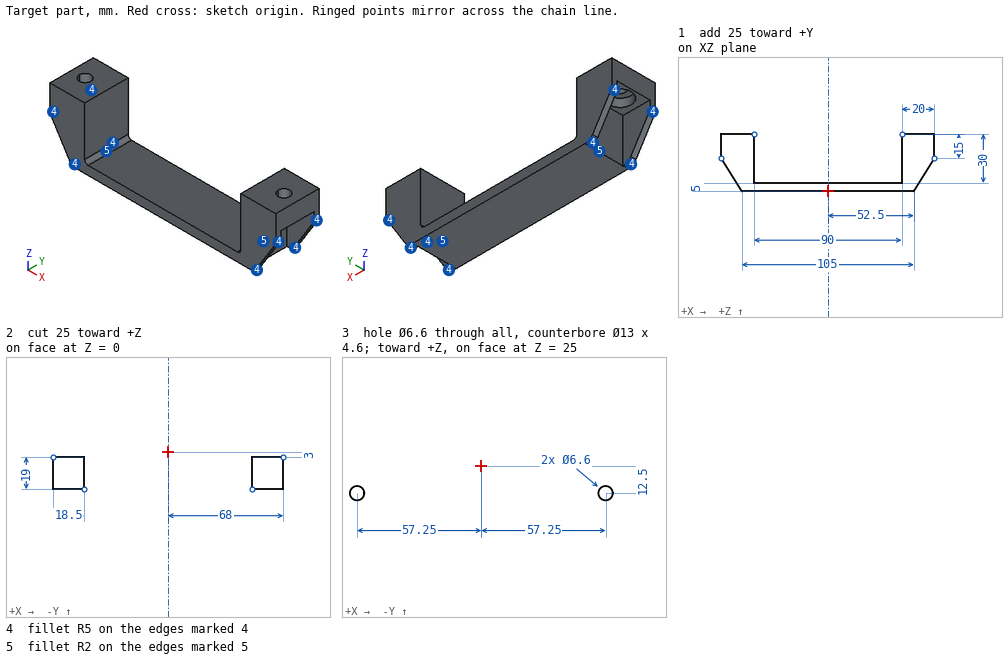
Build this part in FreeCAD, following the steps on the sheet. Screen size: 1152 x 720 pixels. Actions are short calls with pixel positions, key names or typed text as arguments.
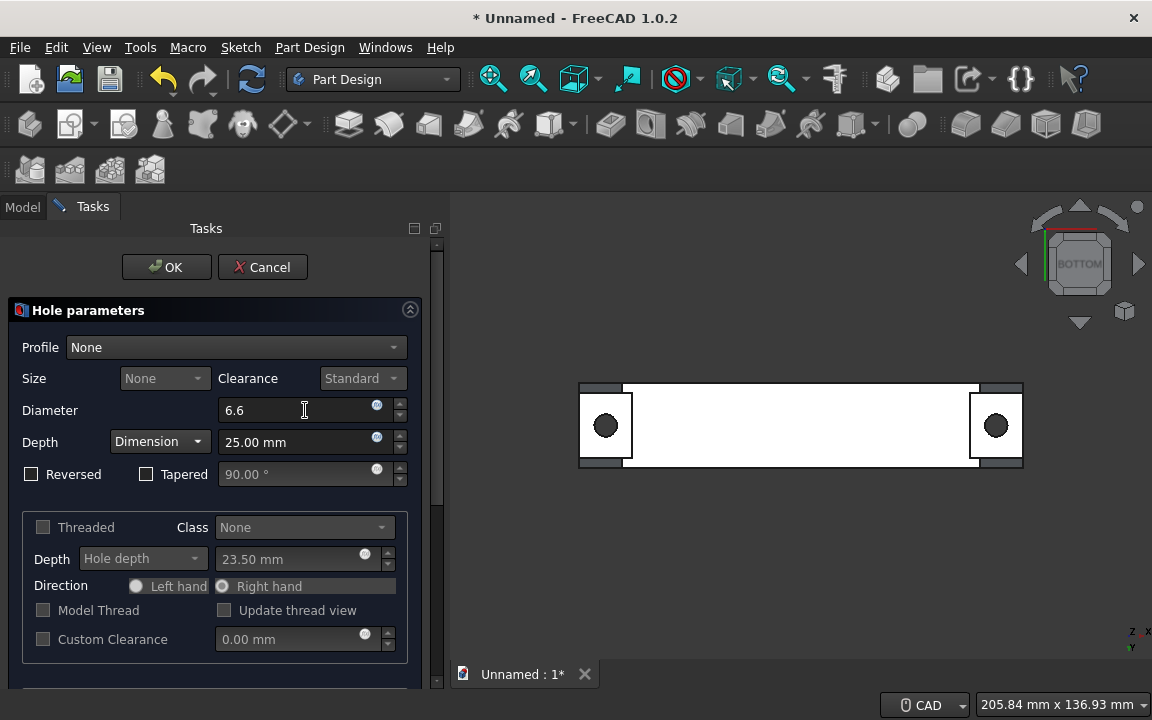
click(161, 442)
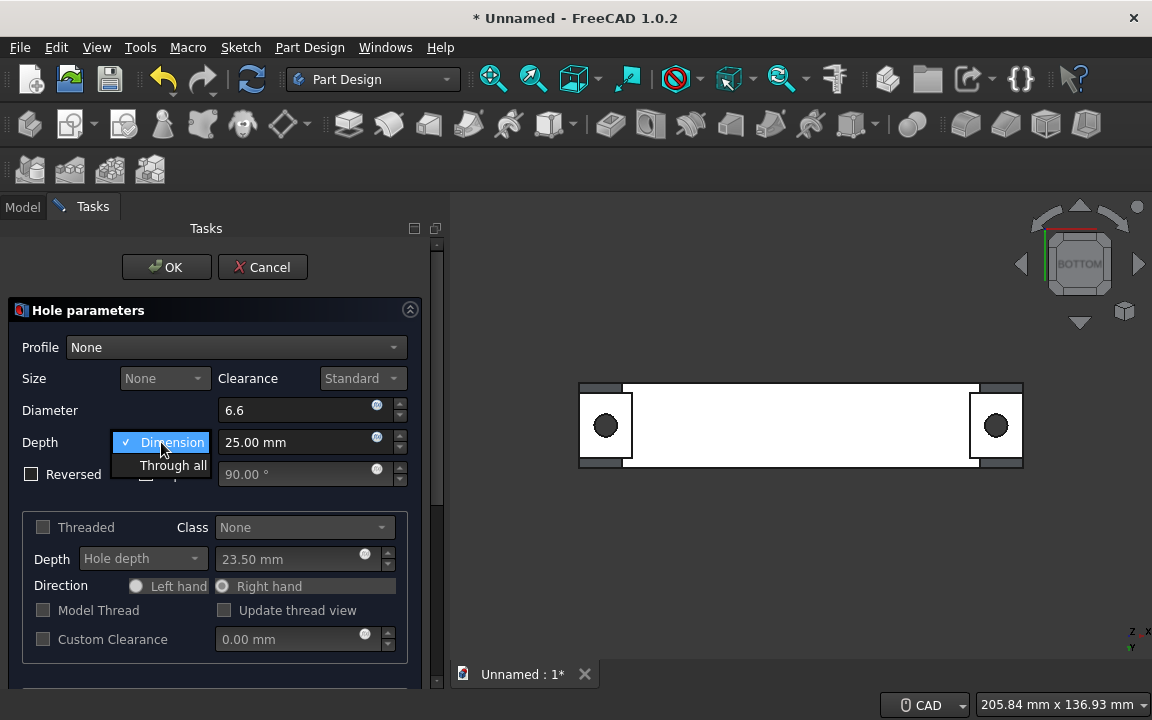
click(160, 466)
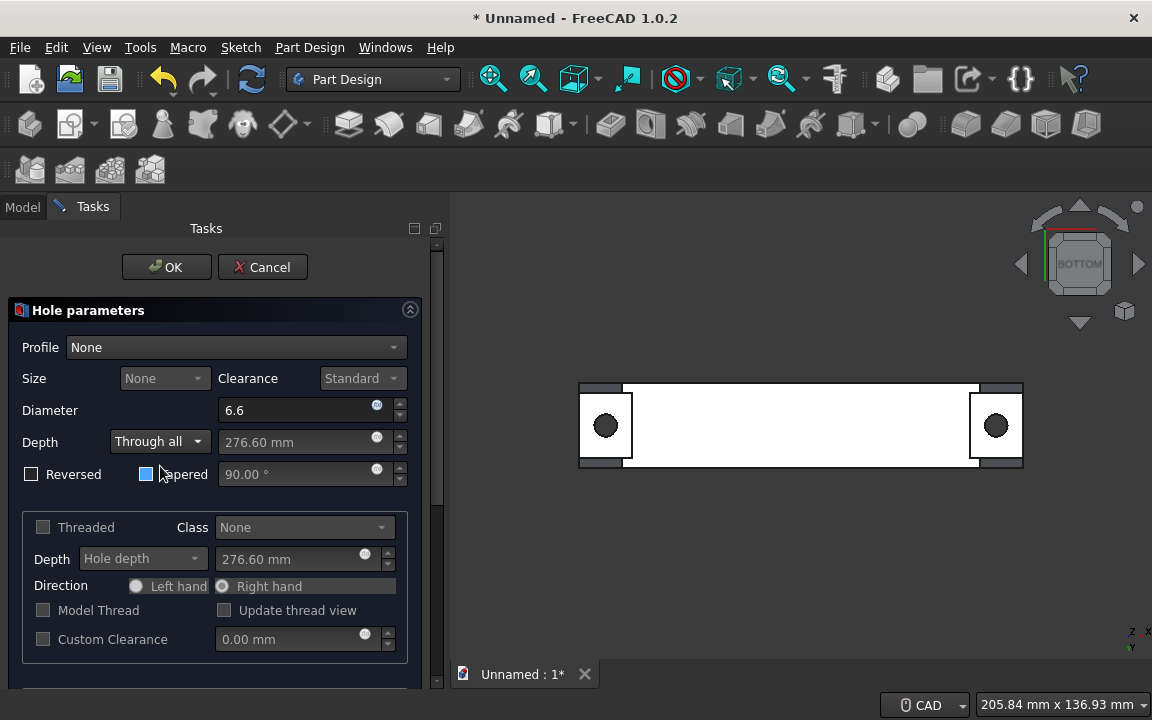
scroll(437, 463, down, 2)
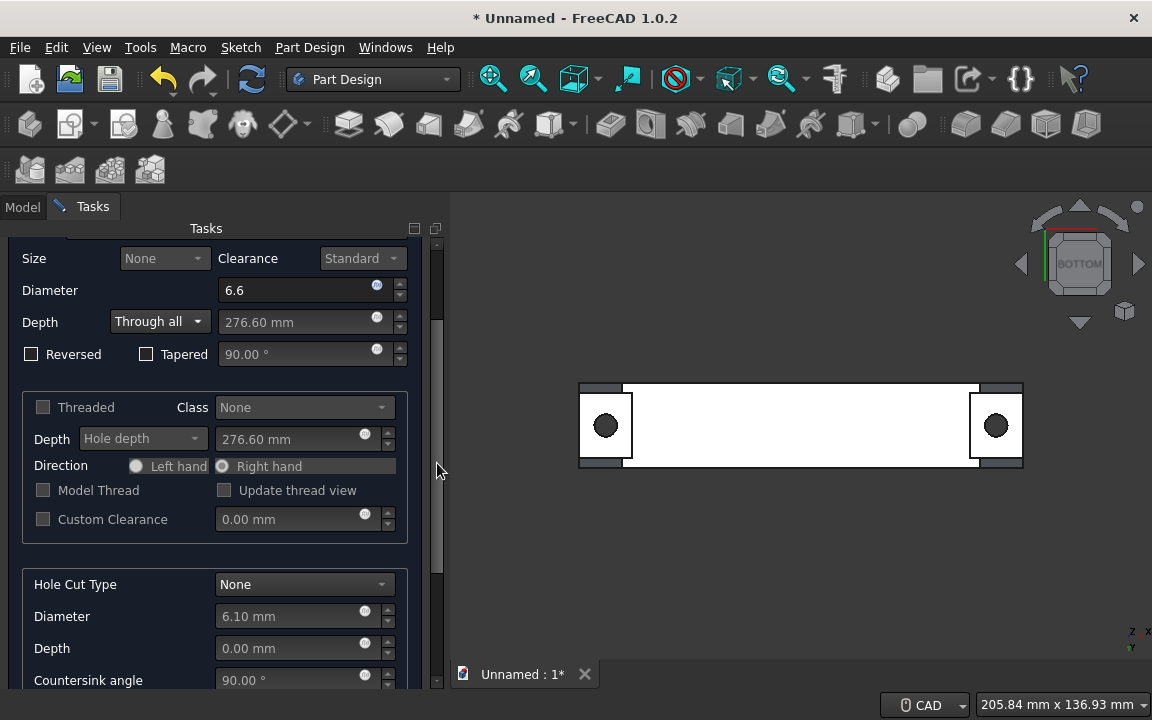
click(306, 584)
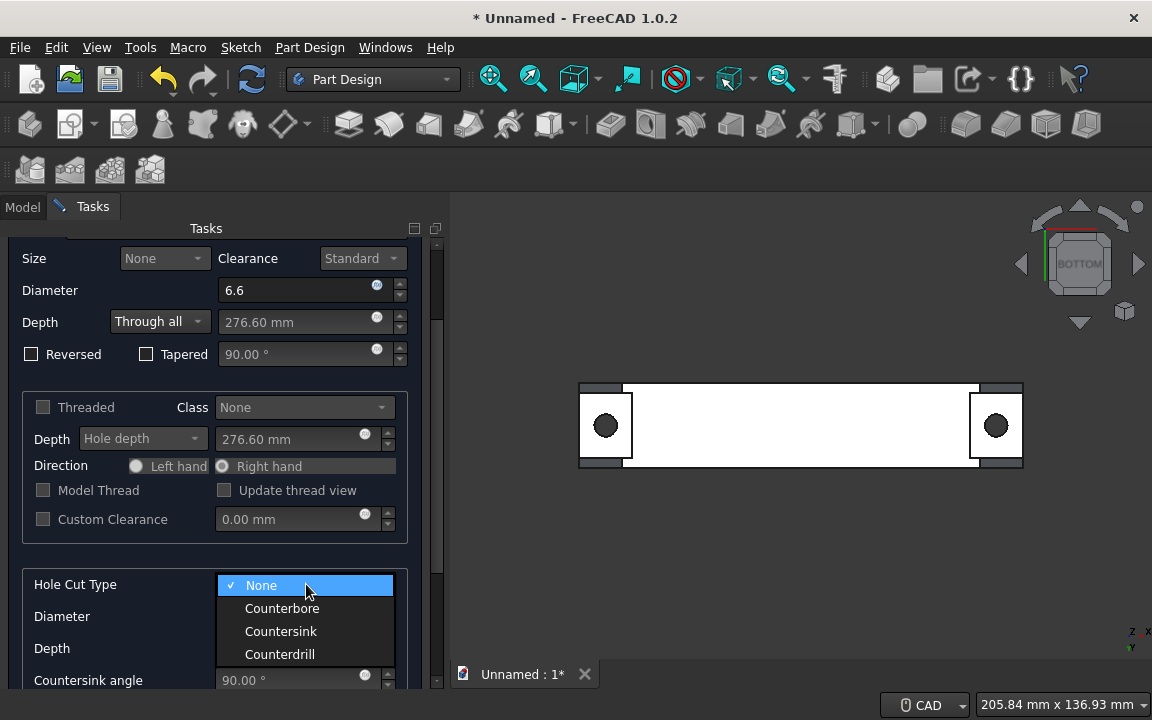
click(304, 608)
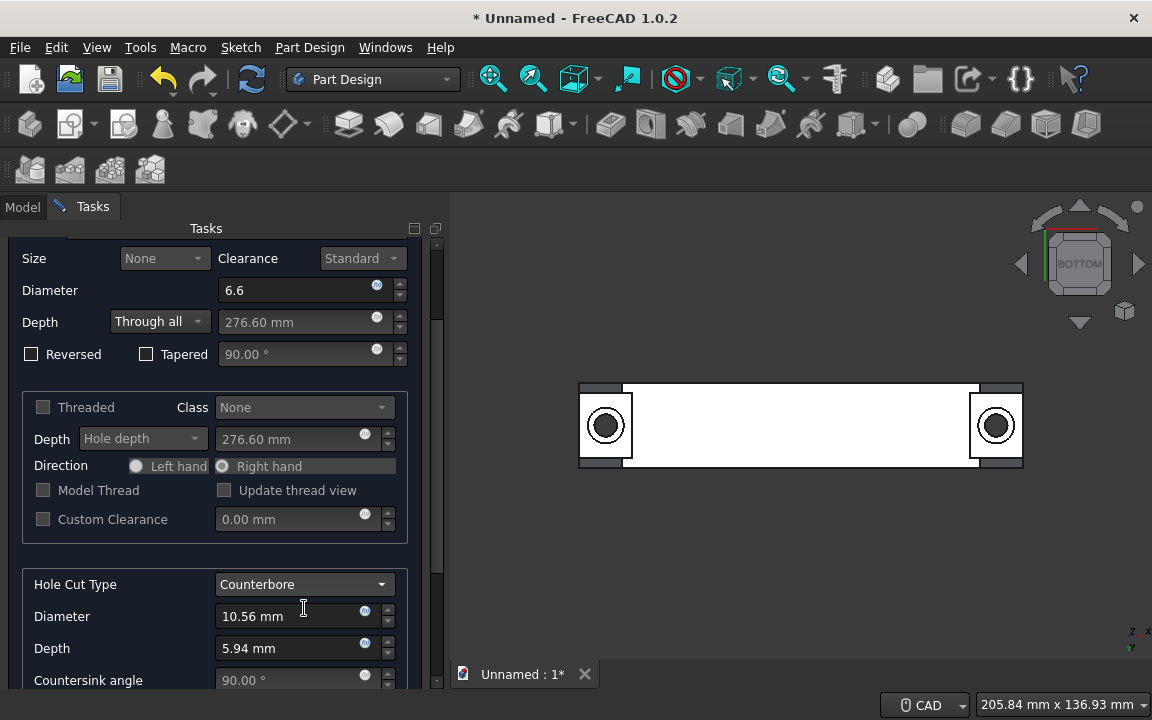
triple_click(298, 616)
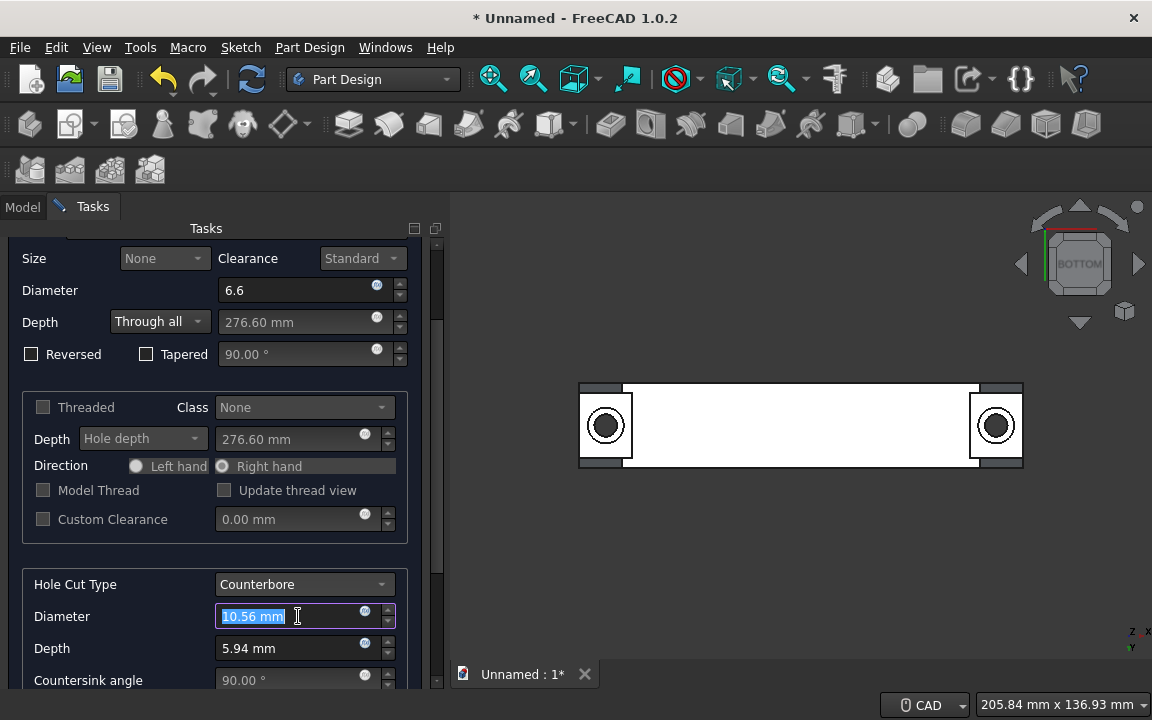
text(13)
key(Tab)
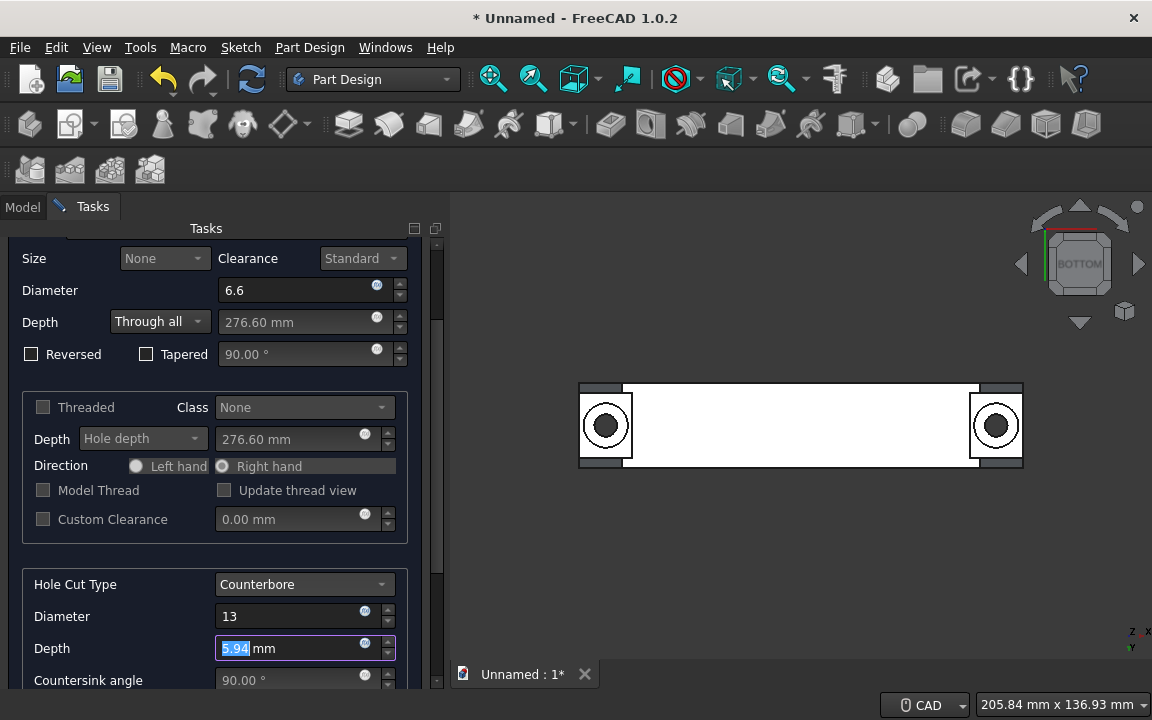
text(4.6)
key(Tab)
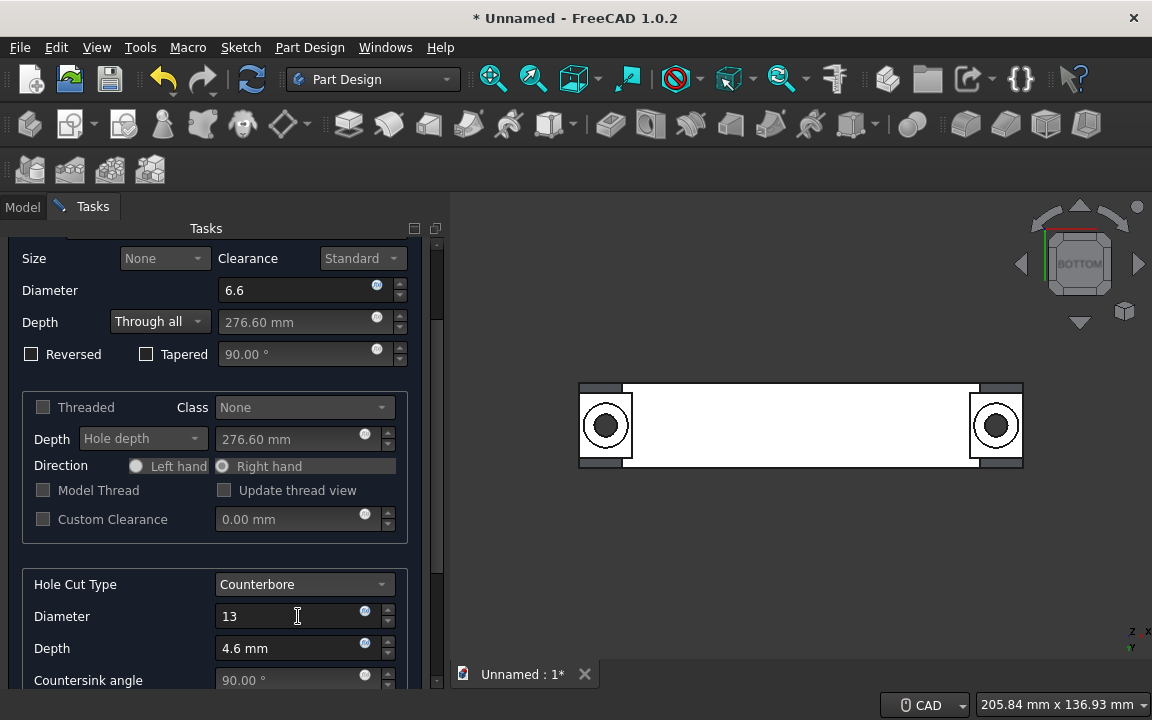
scroll(437, 463, up, 3)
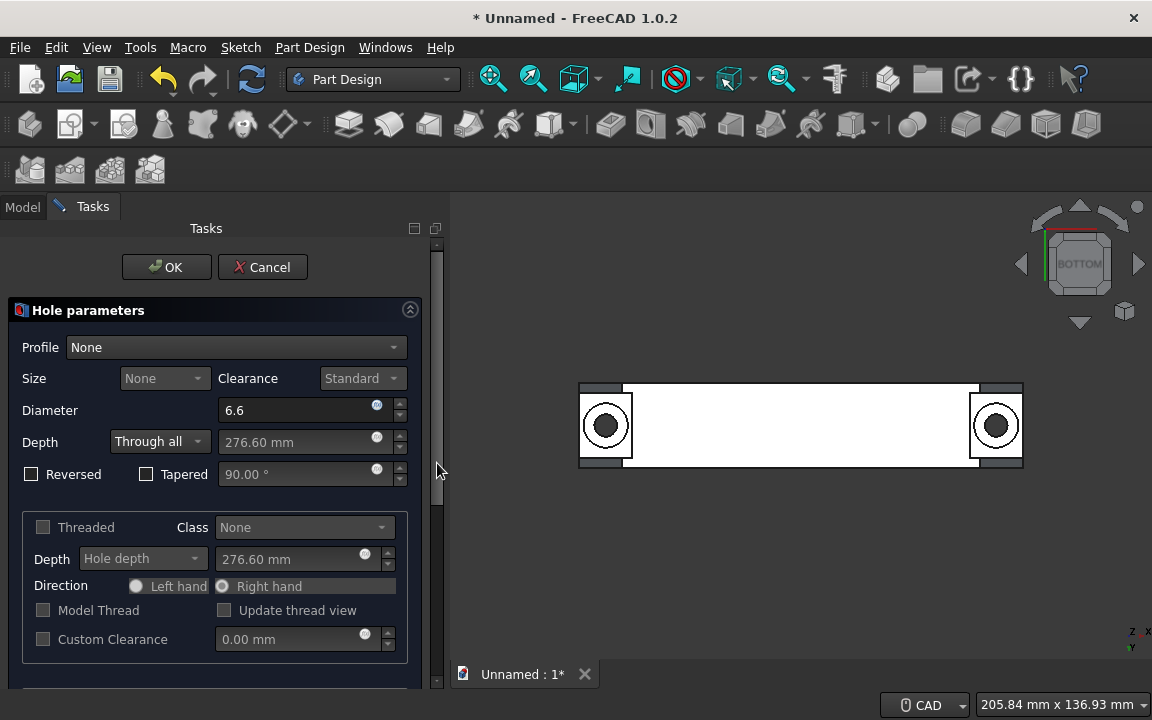
click(167, 267)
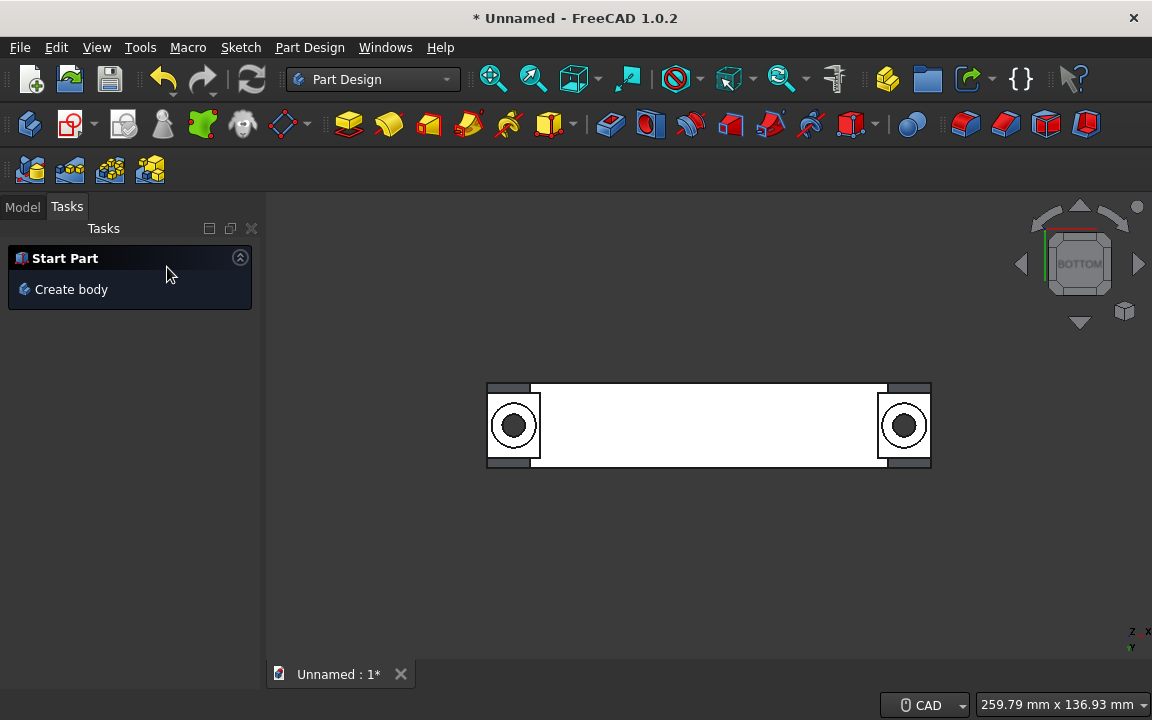
click(530, 463)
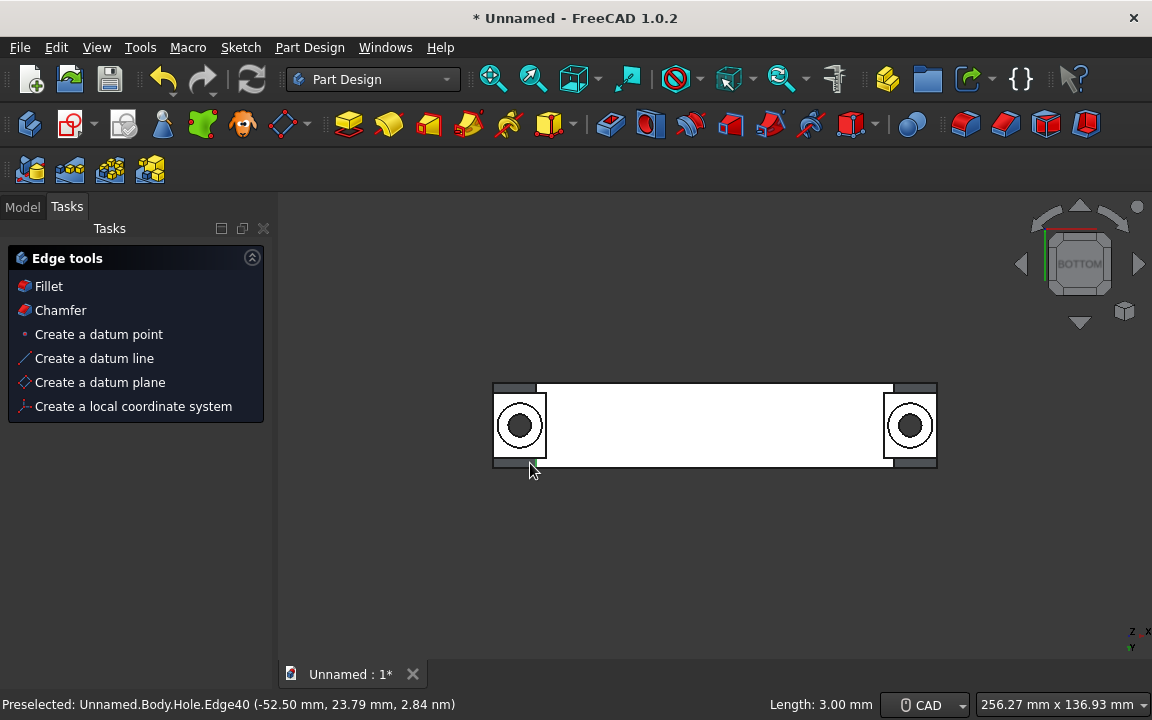
click(894, 463, ctrl)